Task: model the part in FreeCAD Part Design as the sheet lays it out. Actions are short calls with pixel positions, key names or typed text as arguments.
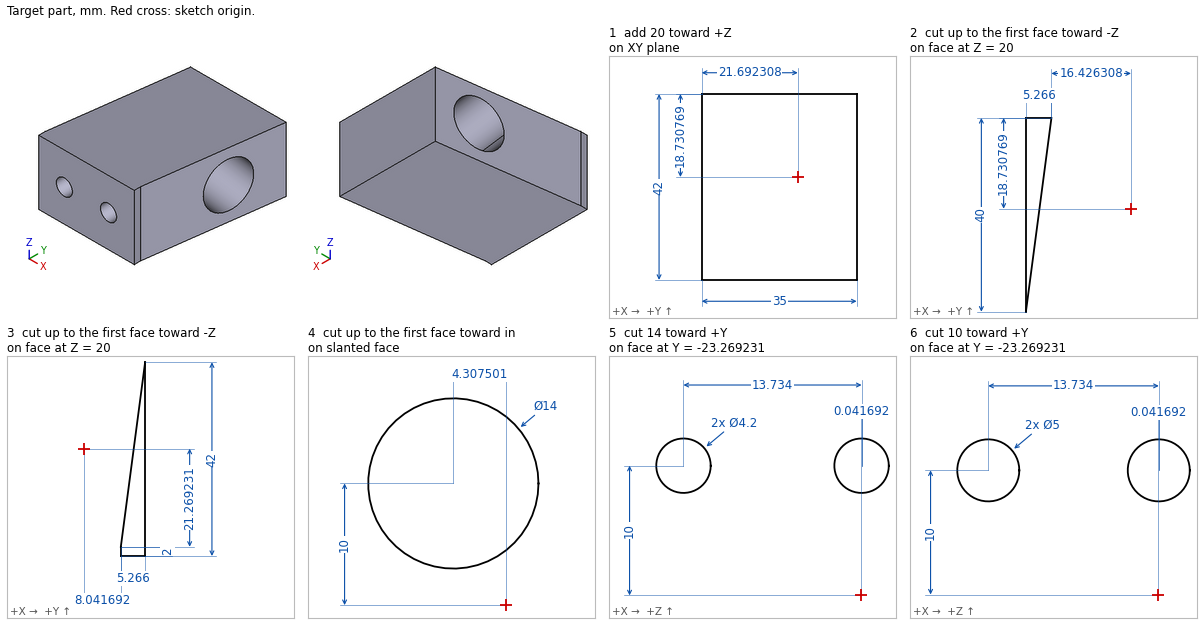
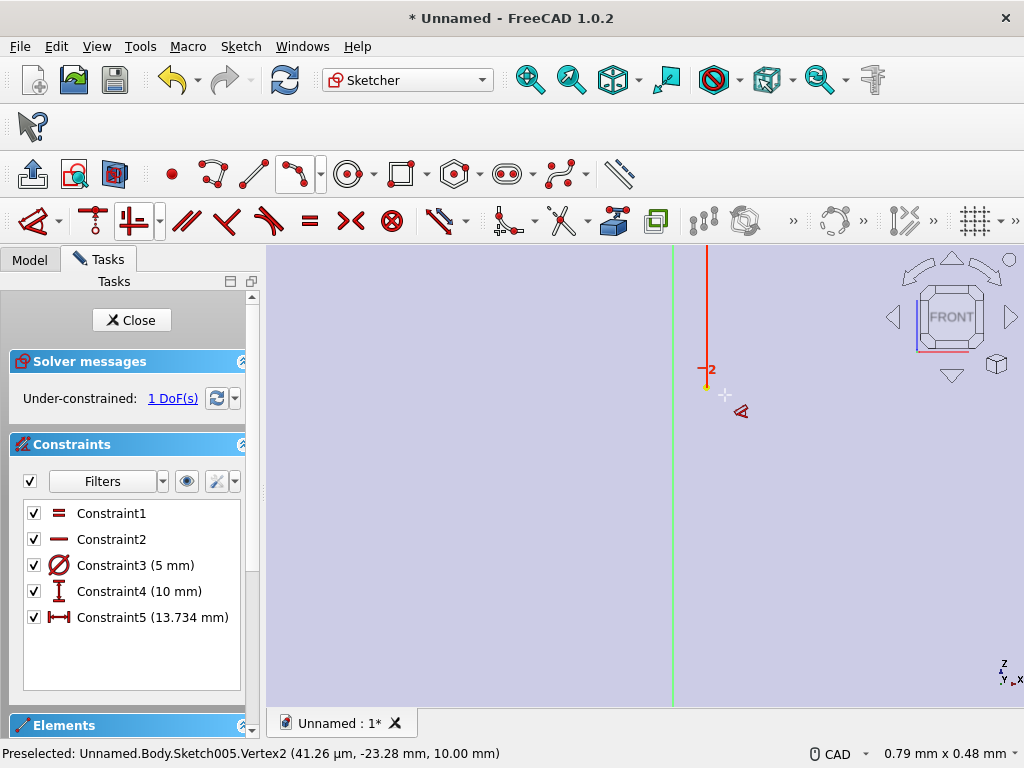
click(707, 388)
click(690, 354)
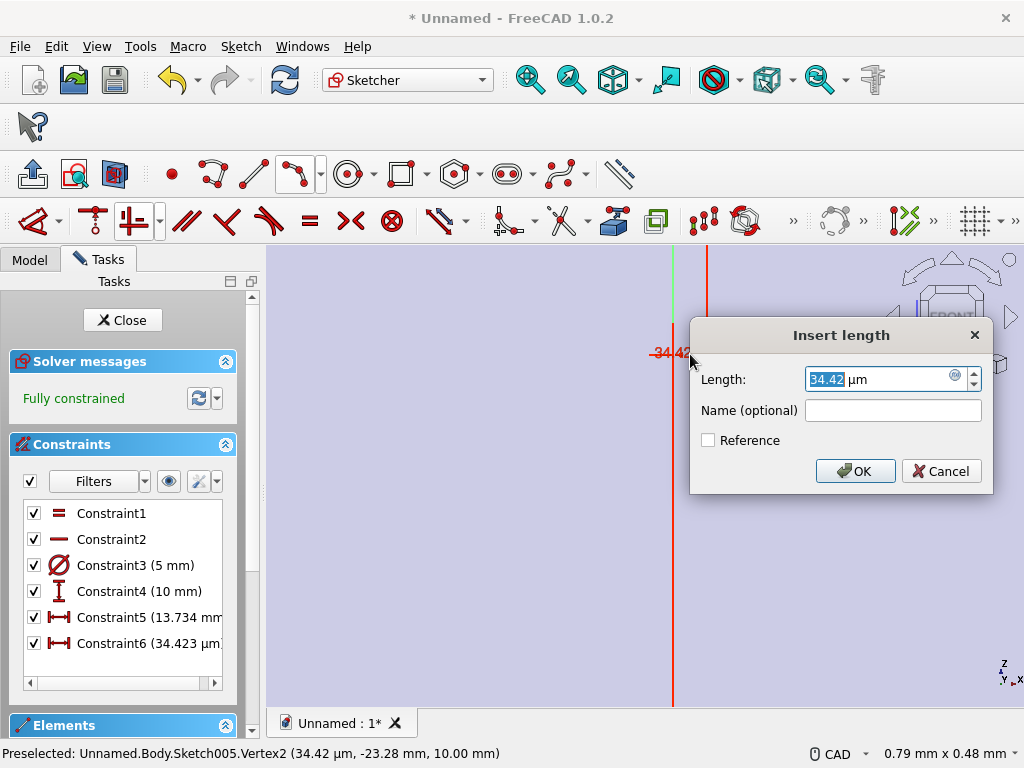
key(ctrl+a)
text(0.041692 mm)
key(Return)
key(Escape)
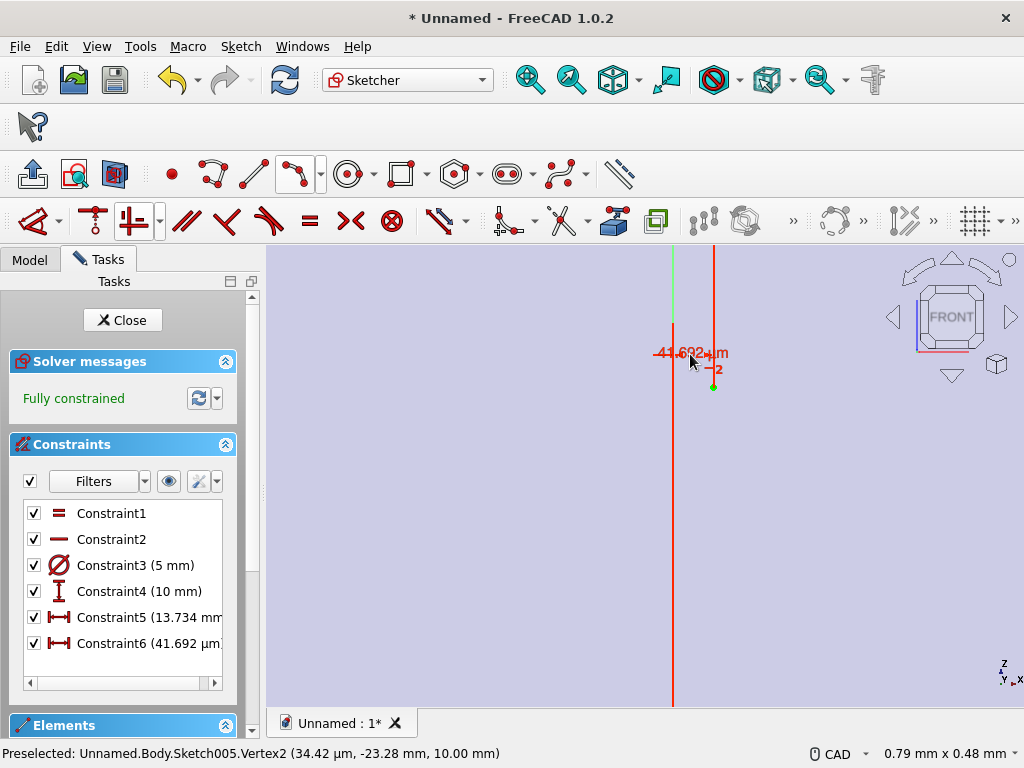
click(123, 320)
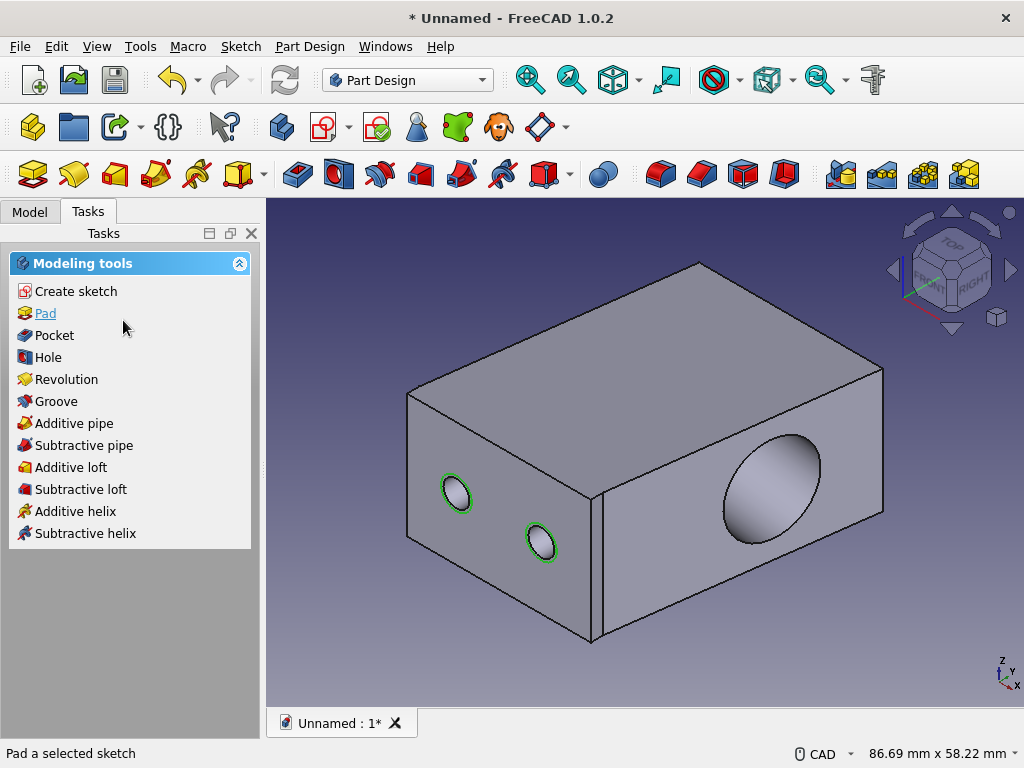
click(298, 174)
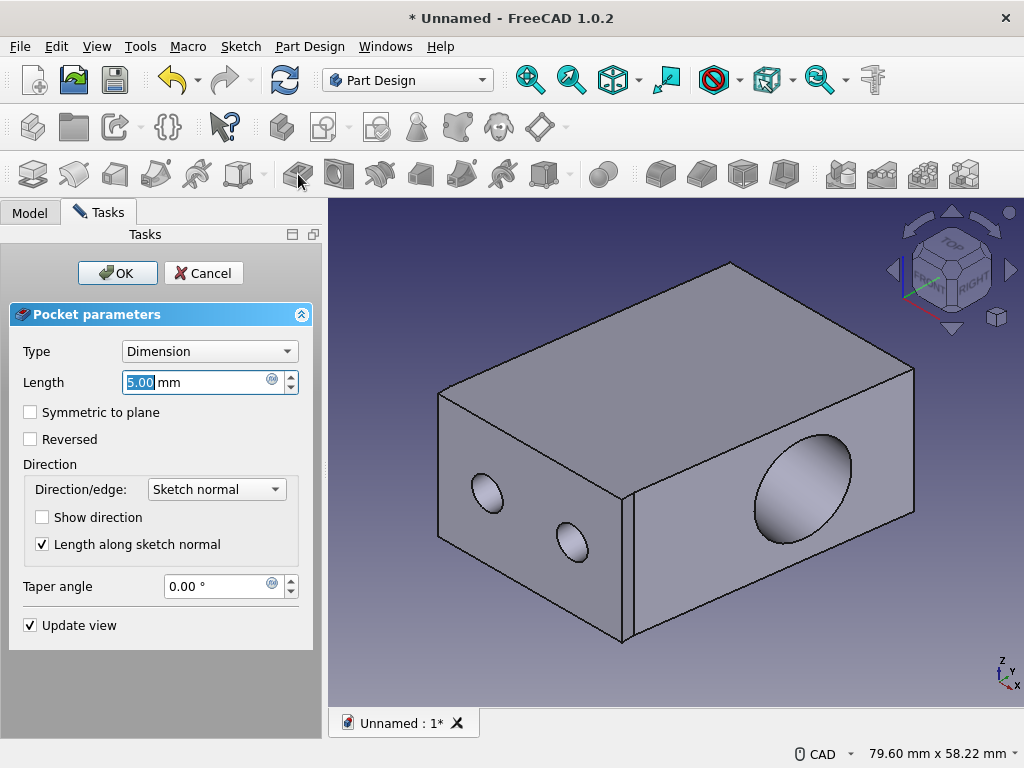
text(10)
key(Tab)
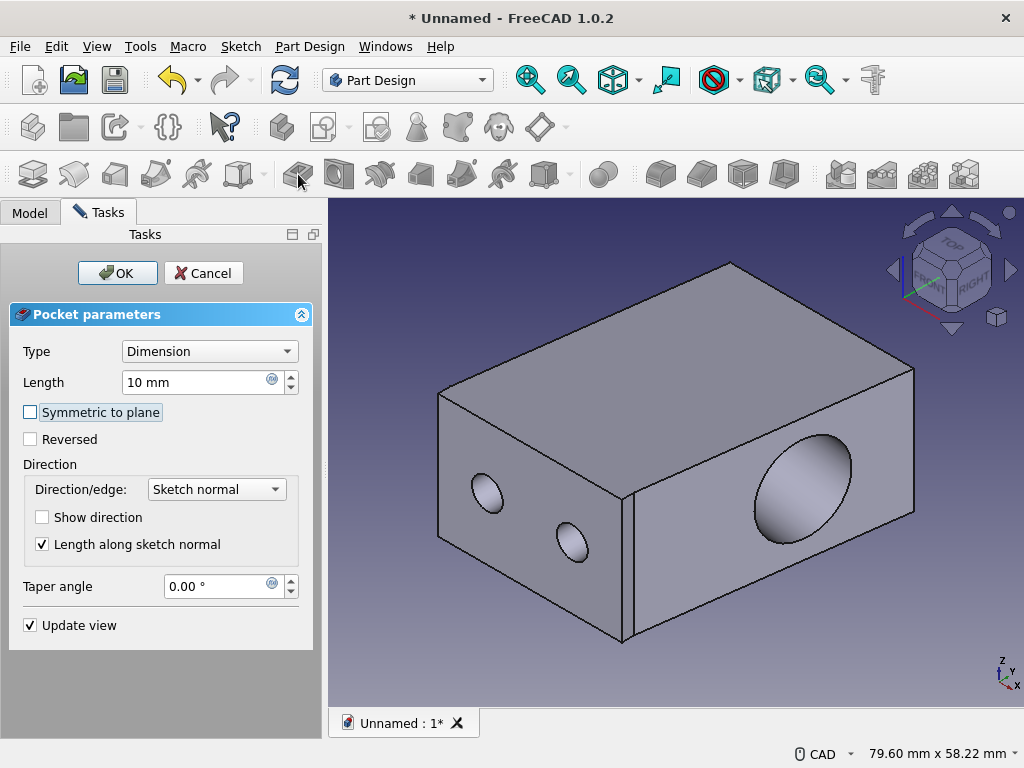
click(118, 273)